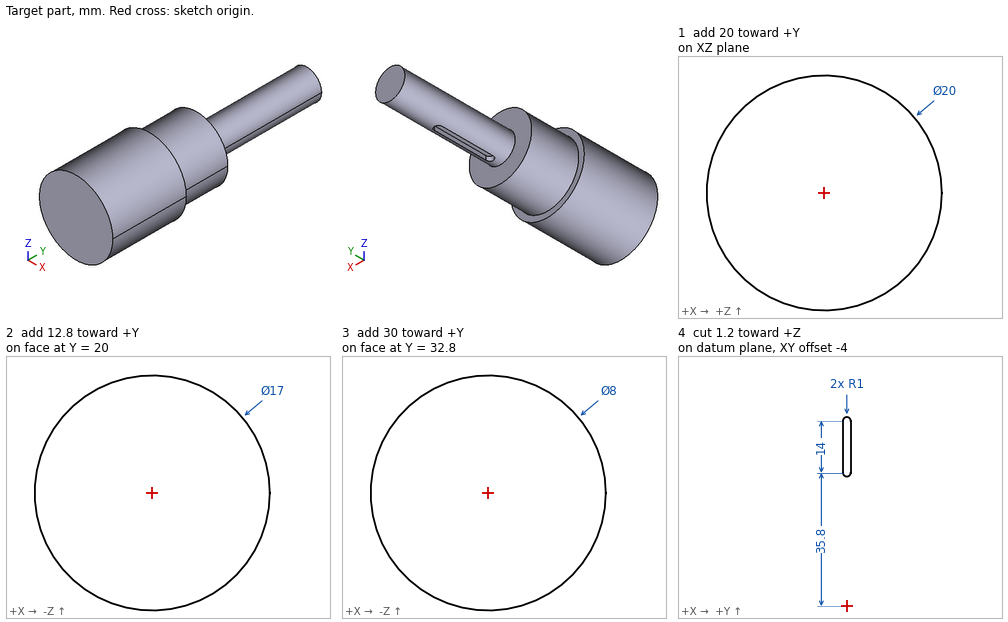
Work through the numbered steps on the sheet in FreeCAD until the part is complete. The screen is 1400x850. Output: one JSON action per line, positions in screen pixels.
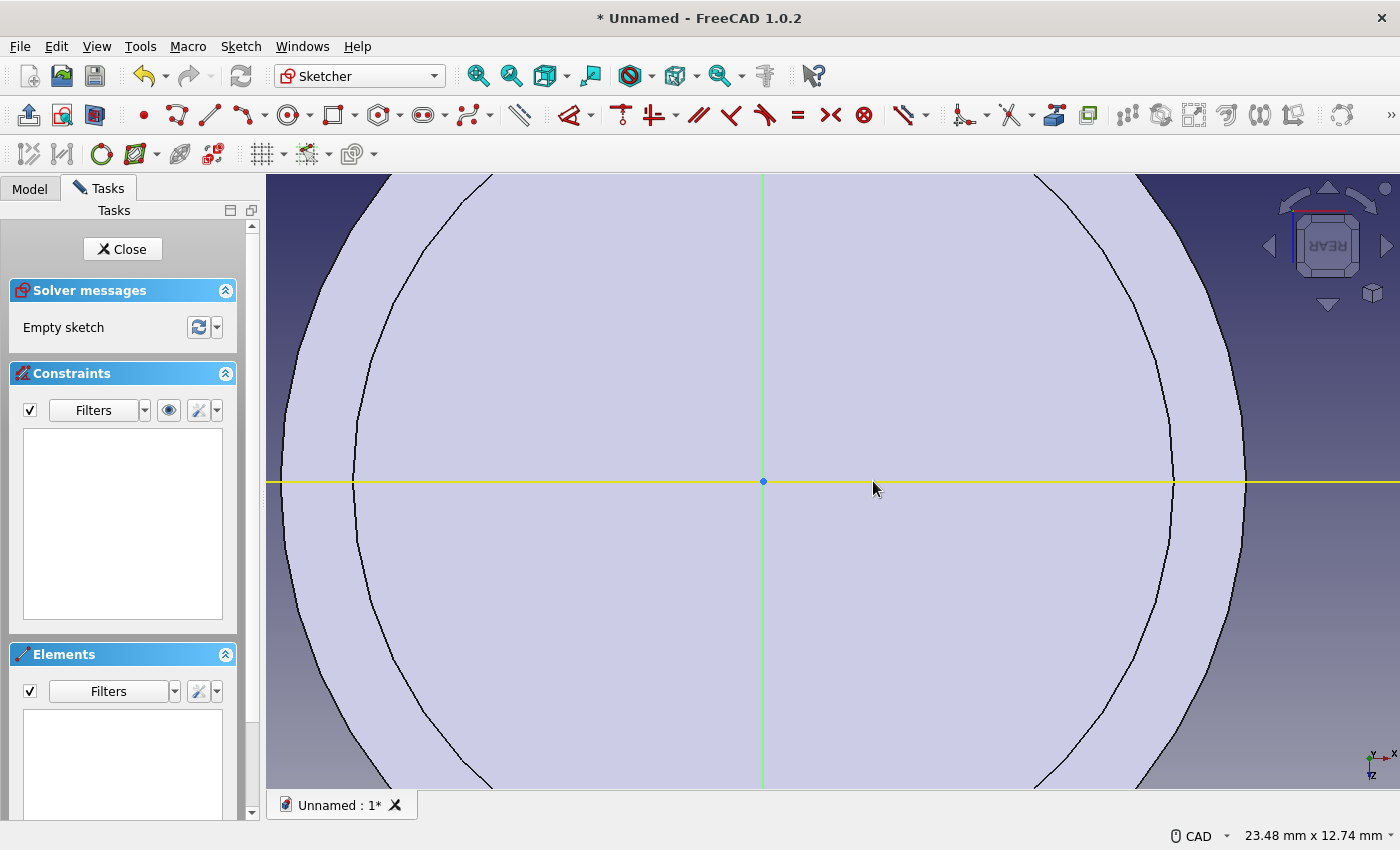
{"action": "left_click", "coordinate": [288, 116]}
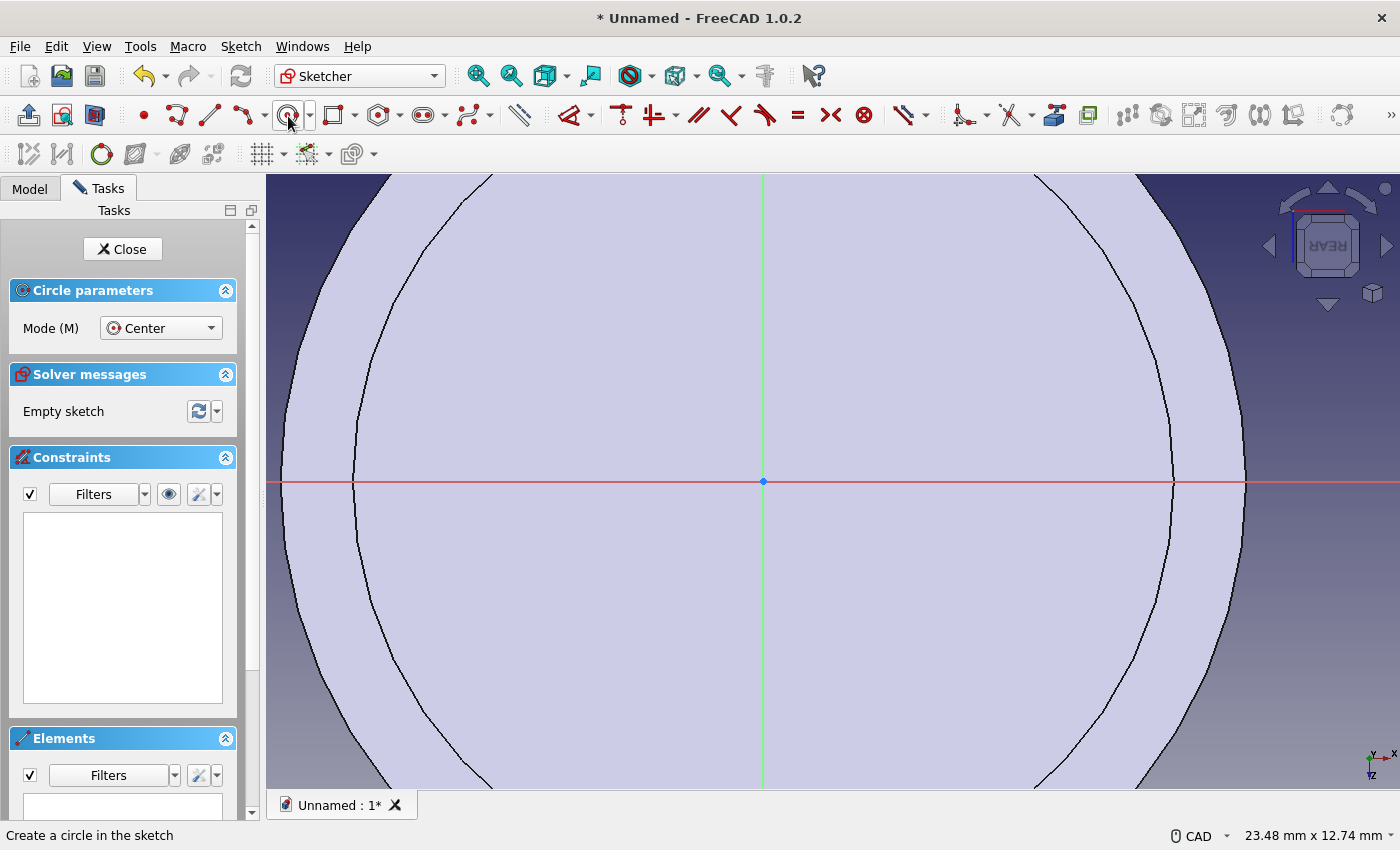
{"action": "left_click", "coordinate": [763, 481]}
{"action": "mouse_move", "coordinate": [900, 345]}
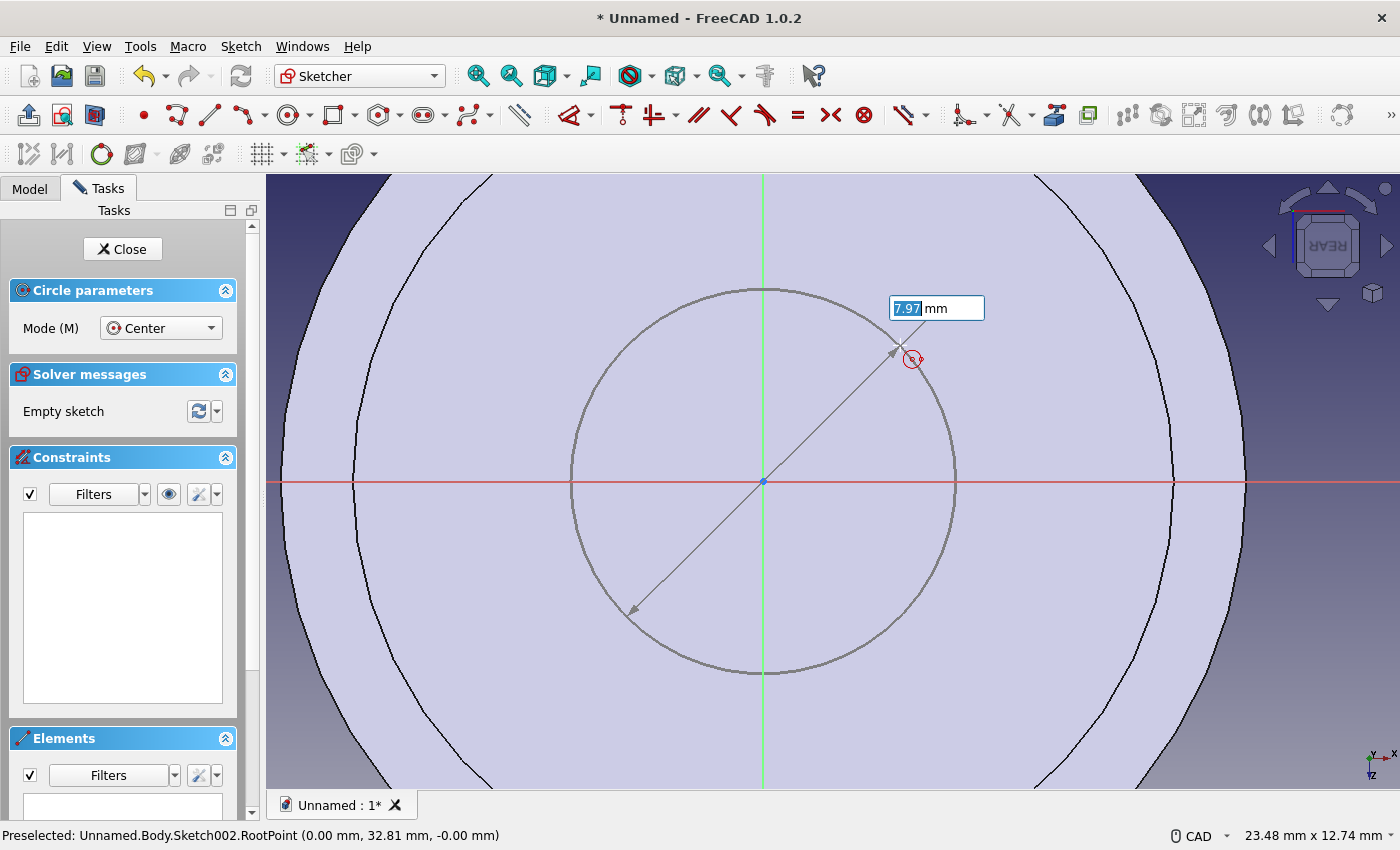
{"action": "type", "text": "8"}
{"action": "key", "text": "Return"}
{"action": "key", "text": "Escape"}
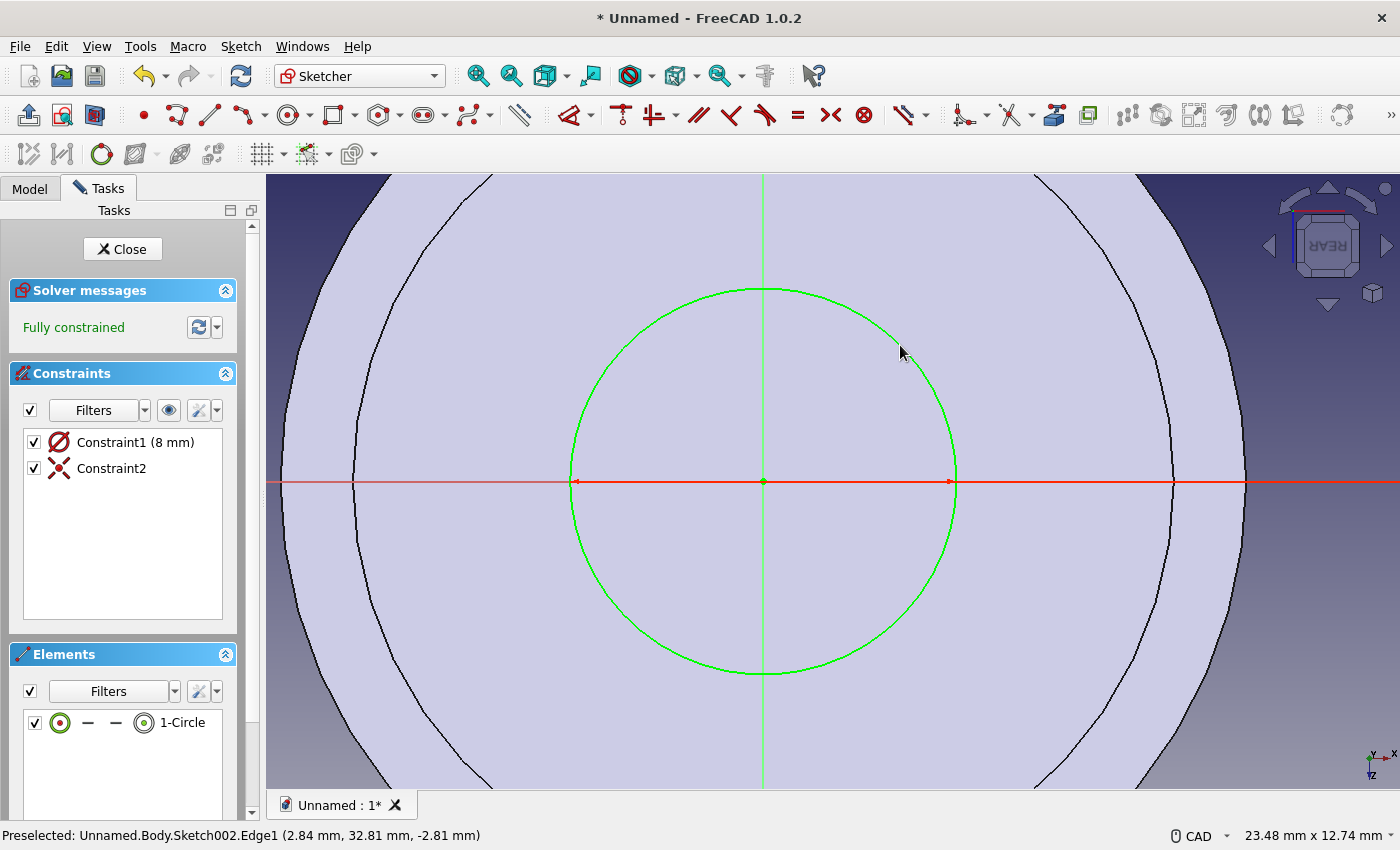
{"action": "left_click", "coordinate": [123, 249]}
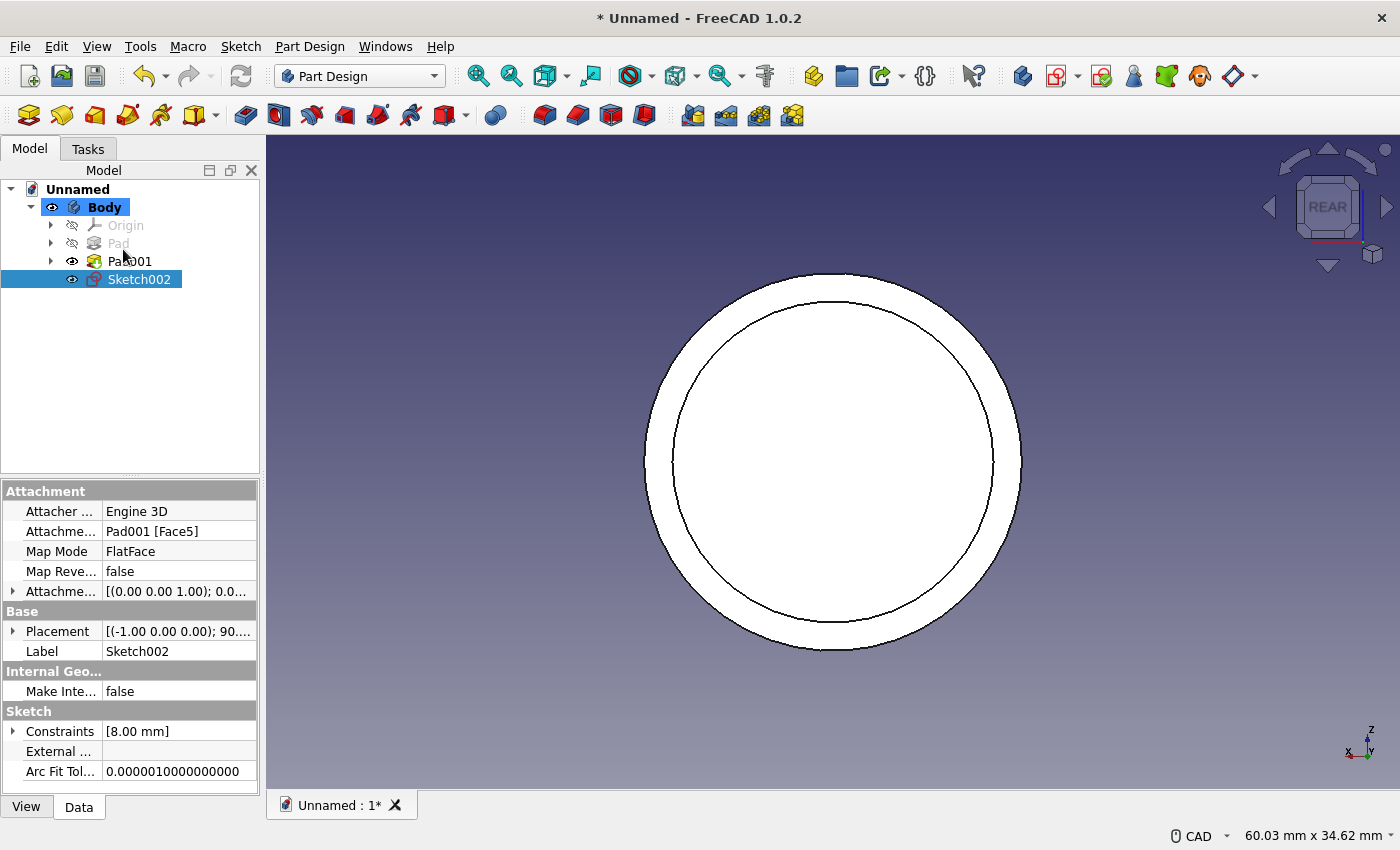
{"action": "left_click", "coordinate": [29, 116]}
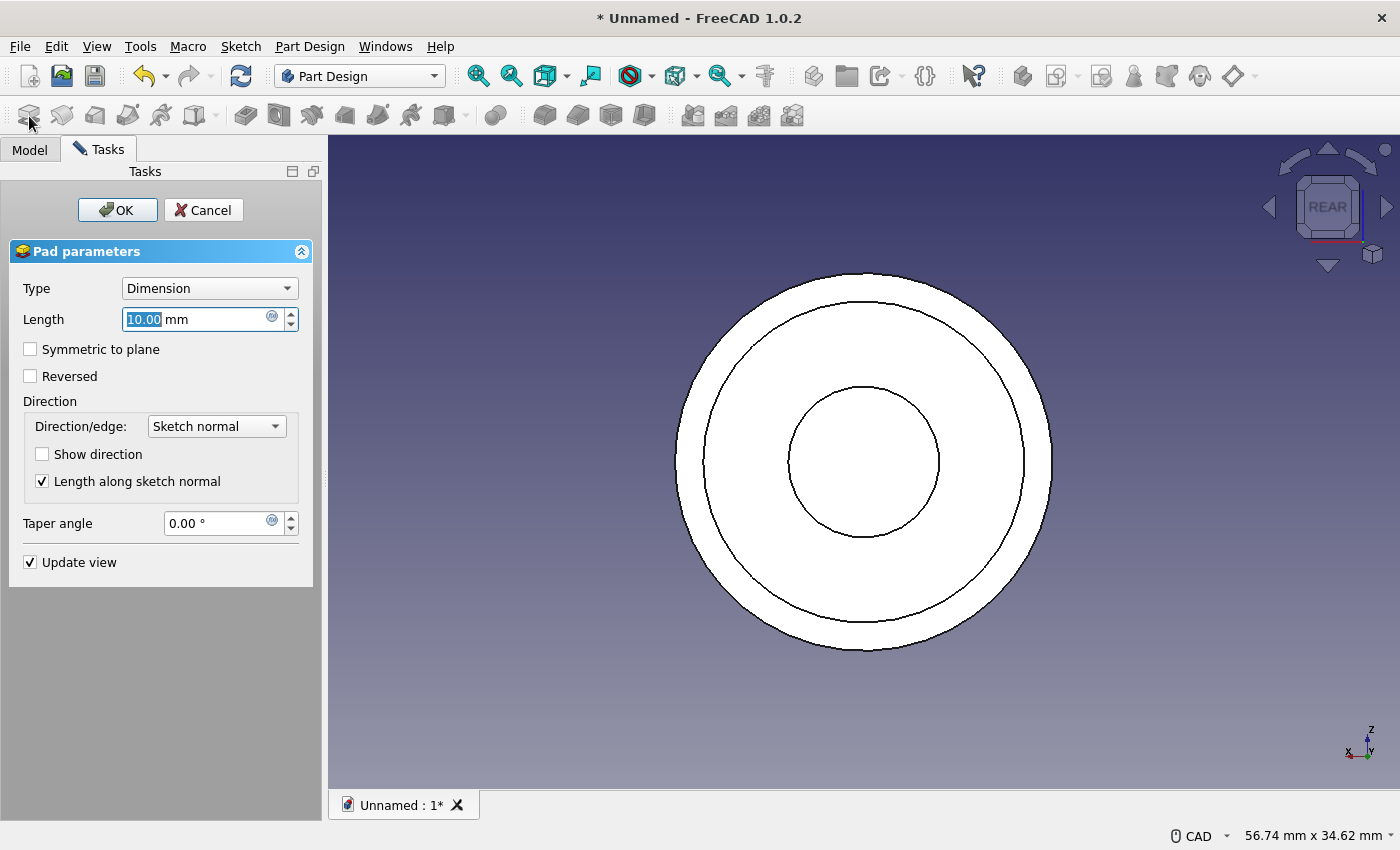
{"action": "type", "text": "30"}
{"action": "key", "text": "Tab"}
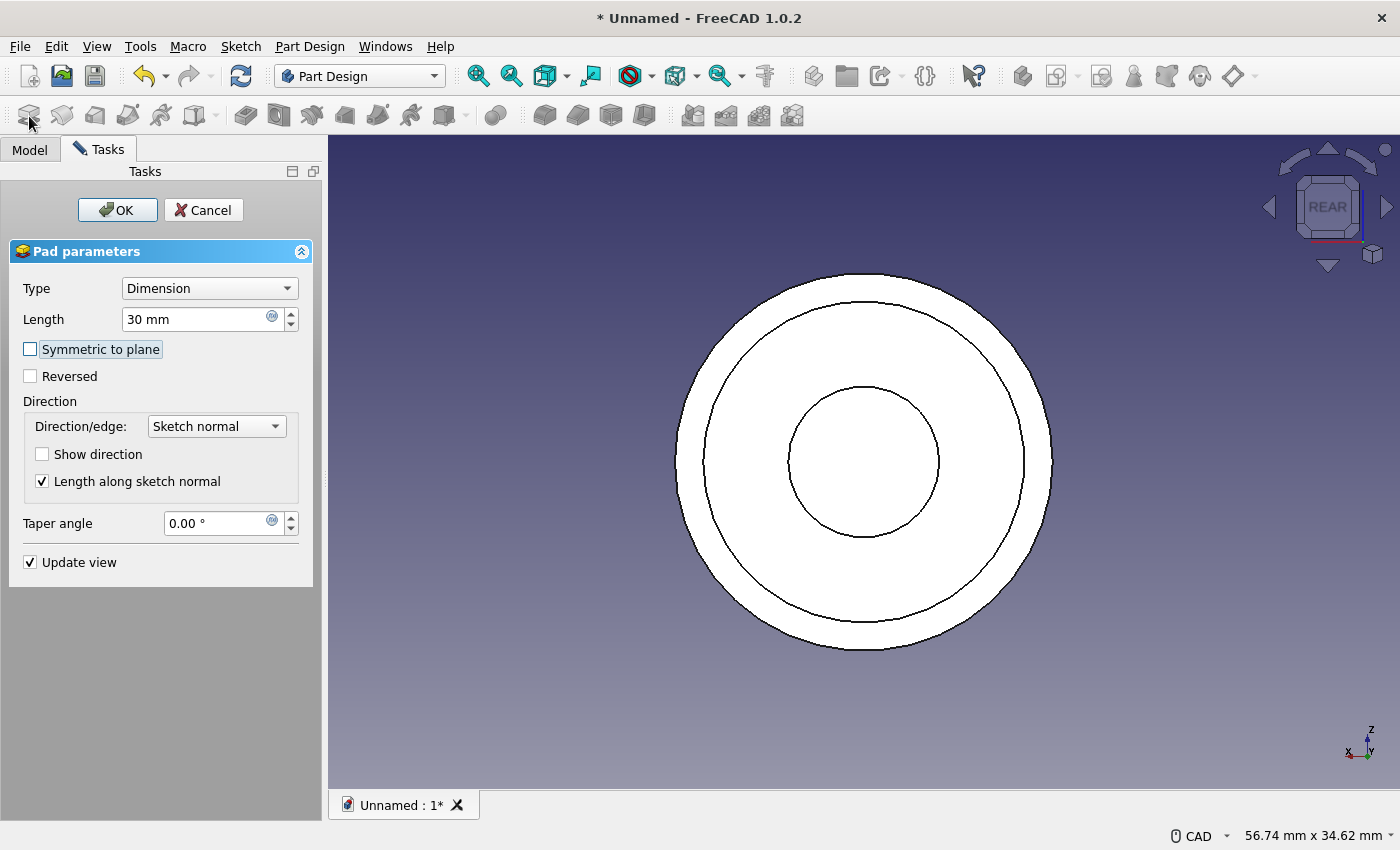
{"action": "left_click", "coordinate": [118, 210]}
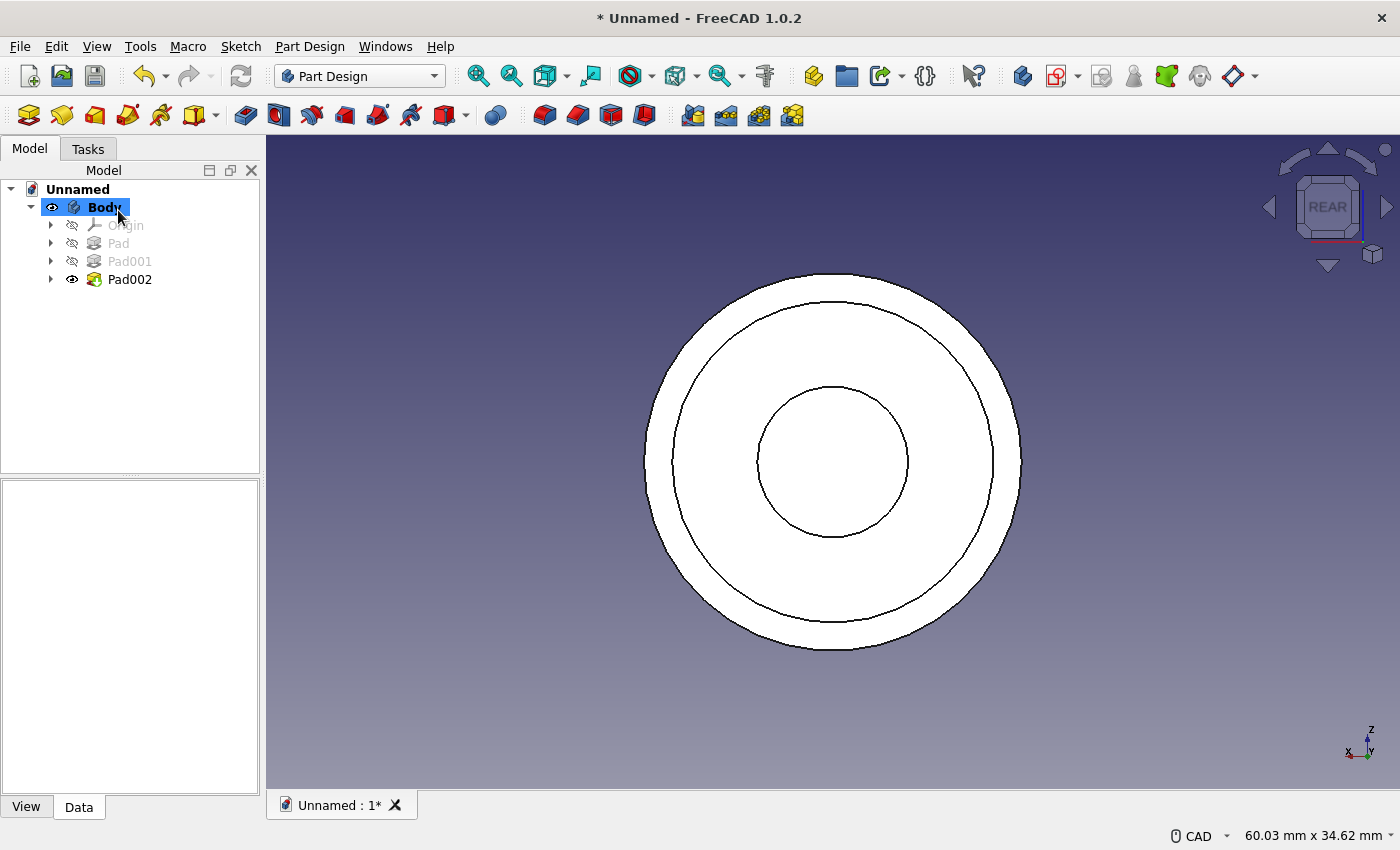
{"action": "left_click", "coordinate": [51, 225]}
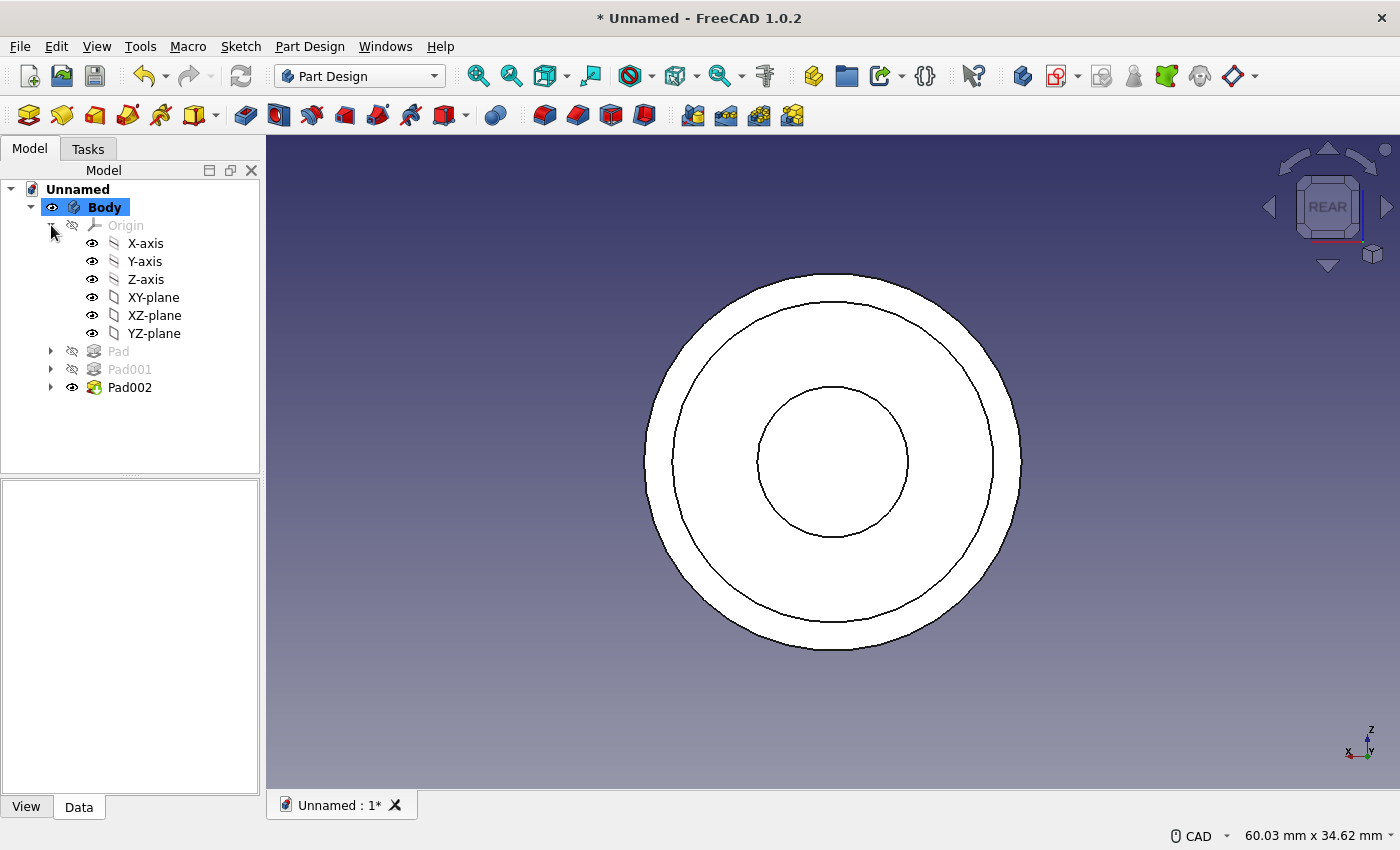
{"action": "left_click", "coordinate": [137, 297]}